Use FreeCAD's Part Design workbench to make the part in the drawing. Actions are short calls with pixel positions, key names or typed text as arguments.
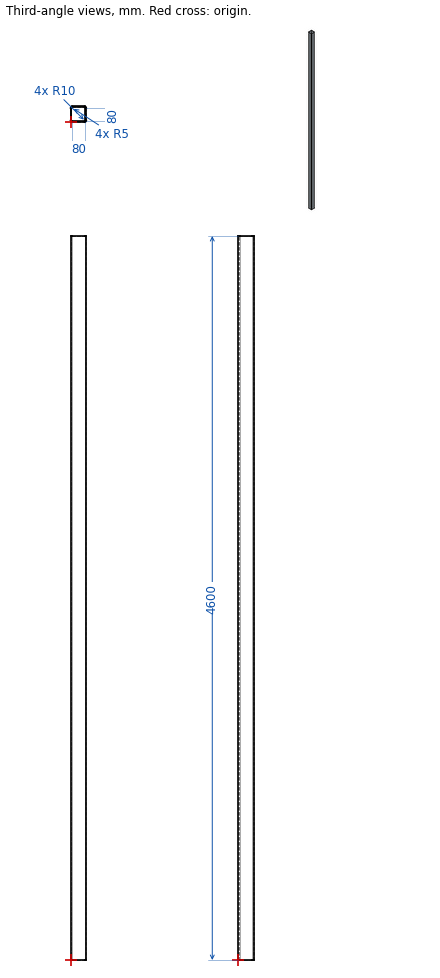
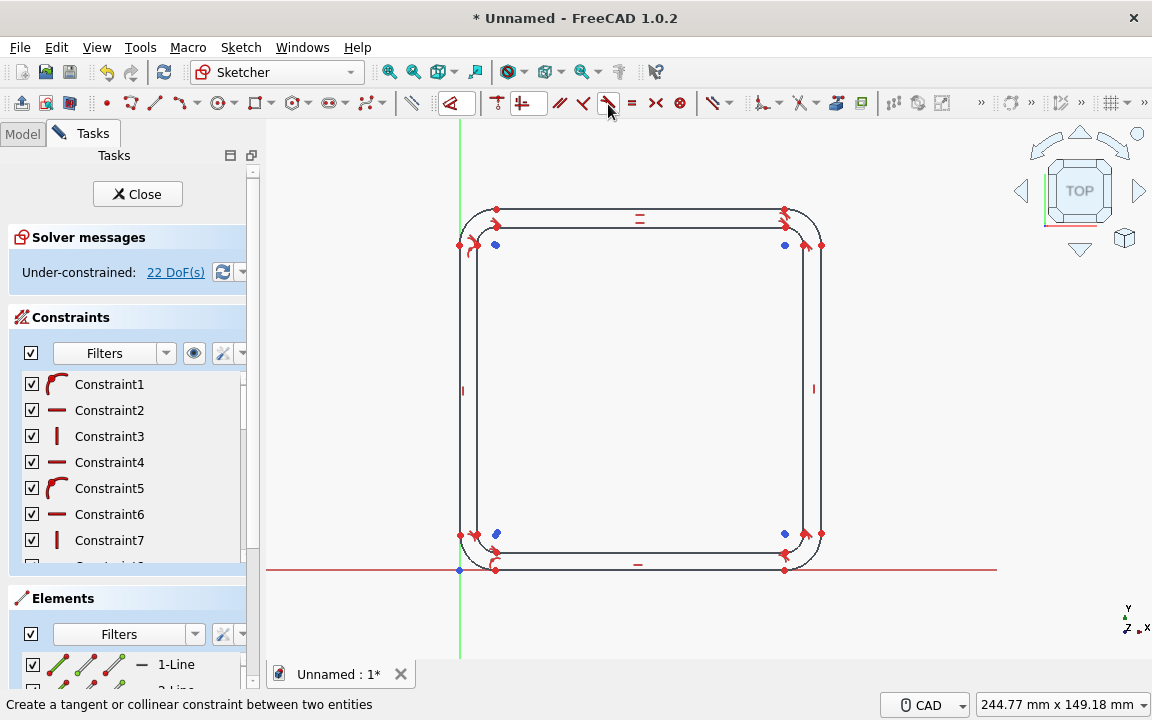
click(583, 228)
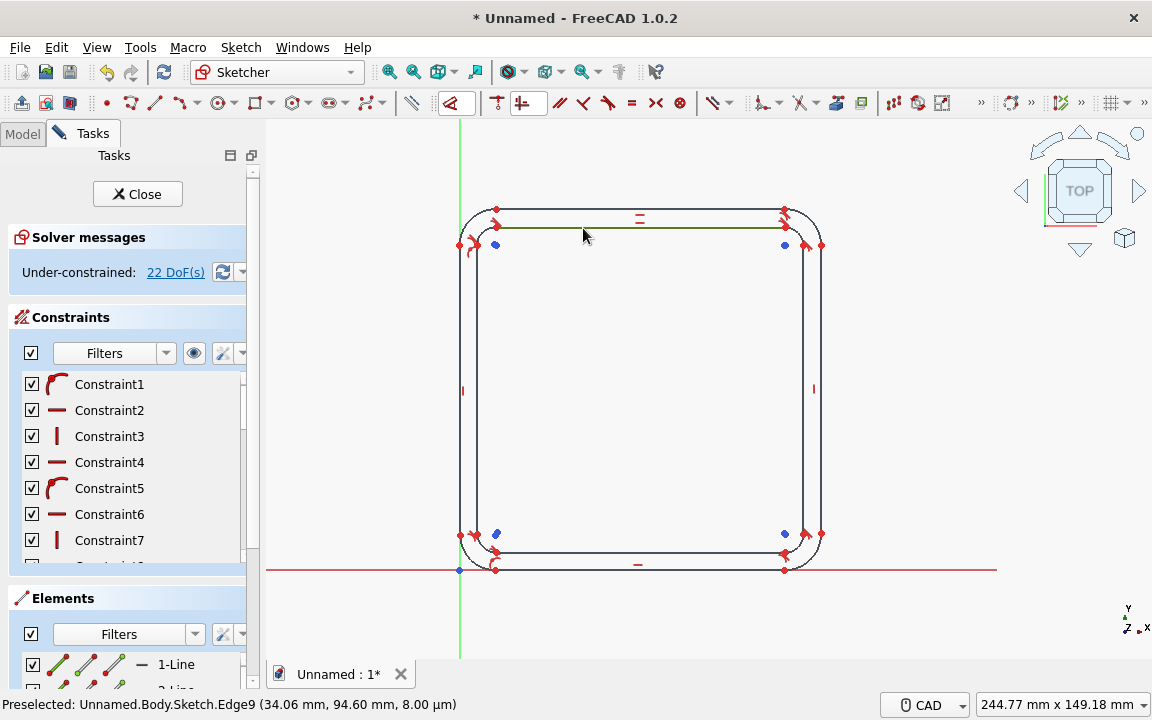
click(483, 232)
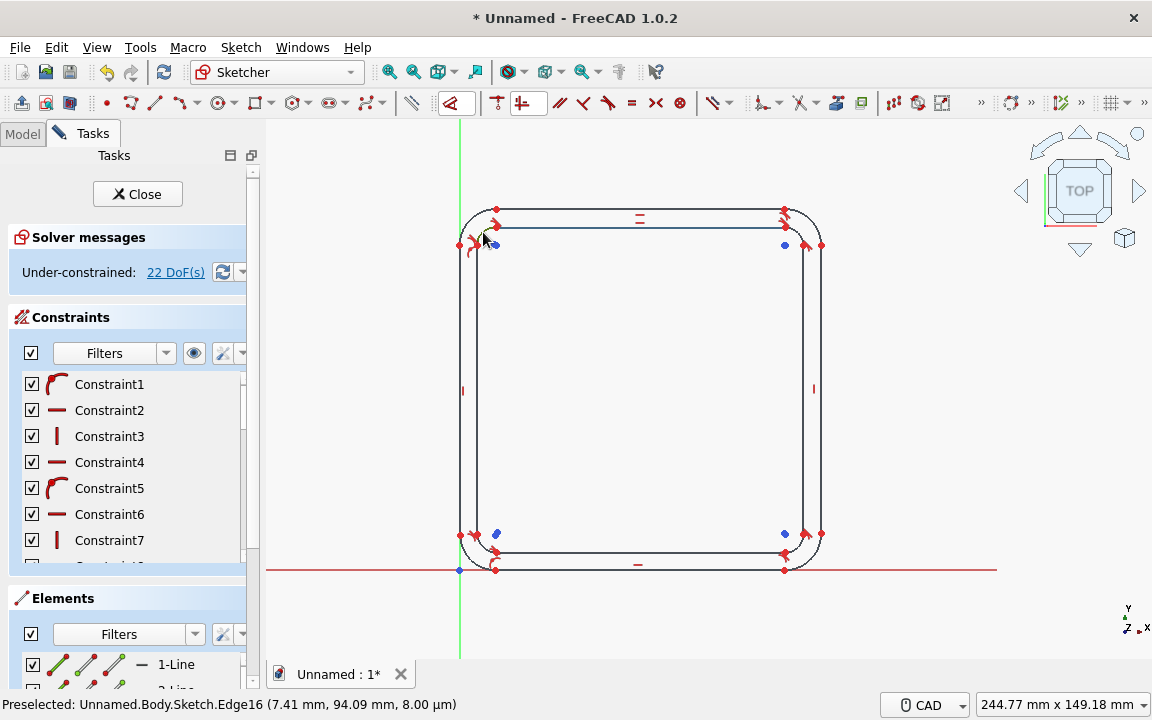
click(608, 104)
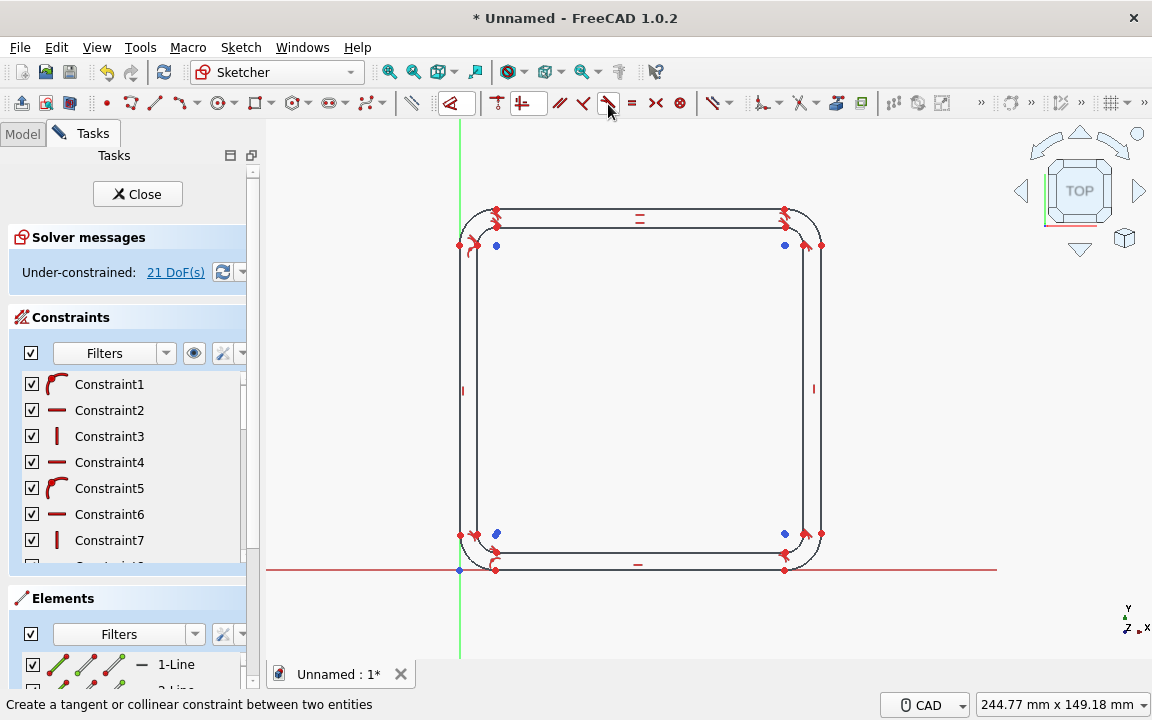
click(803, 332)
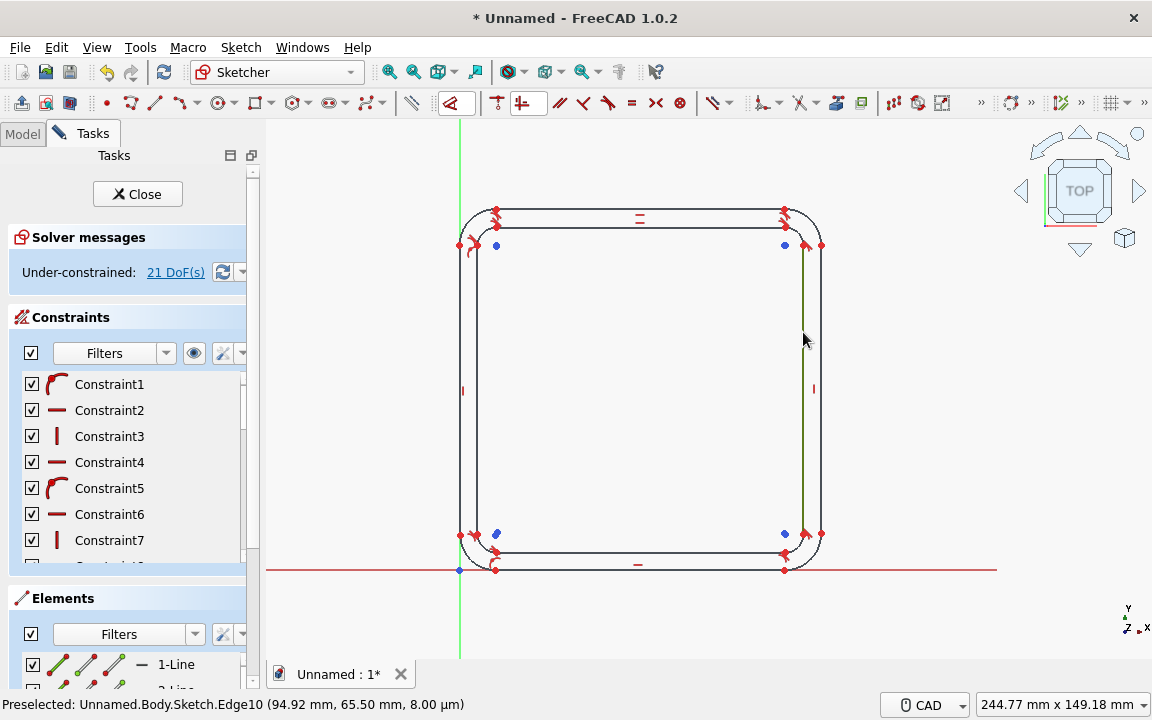
click(798, 233)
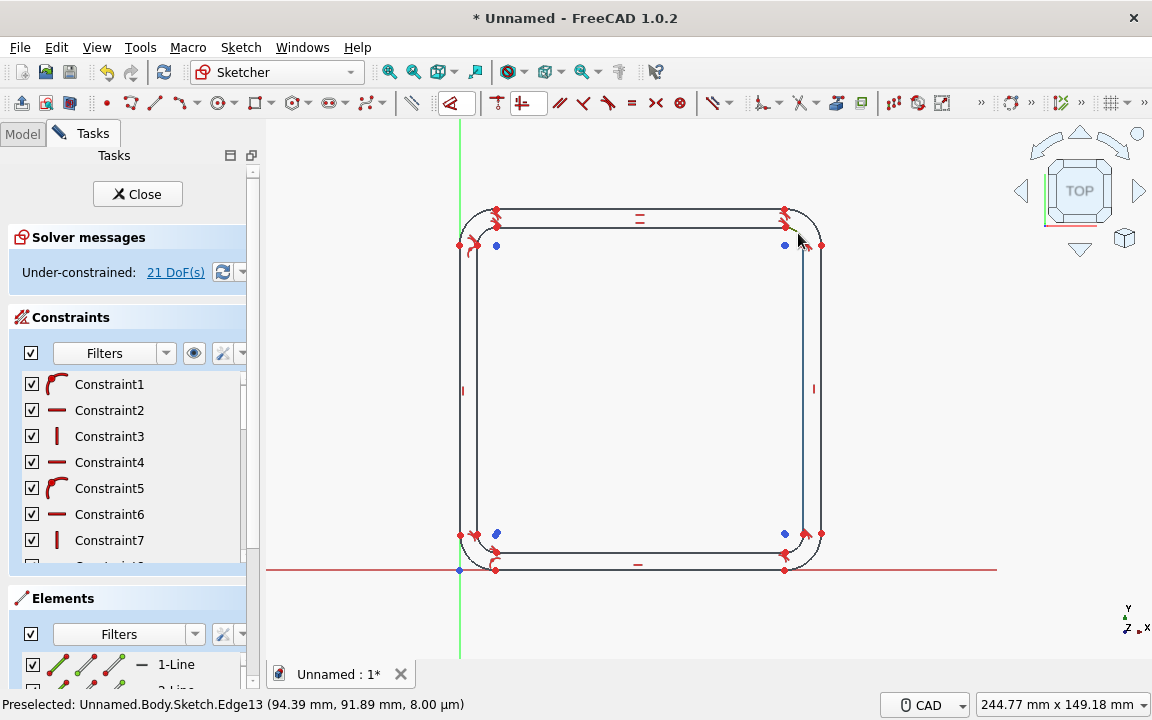
click(608, 104)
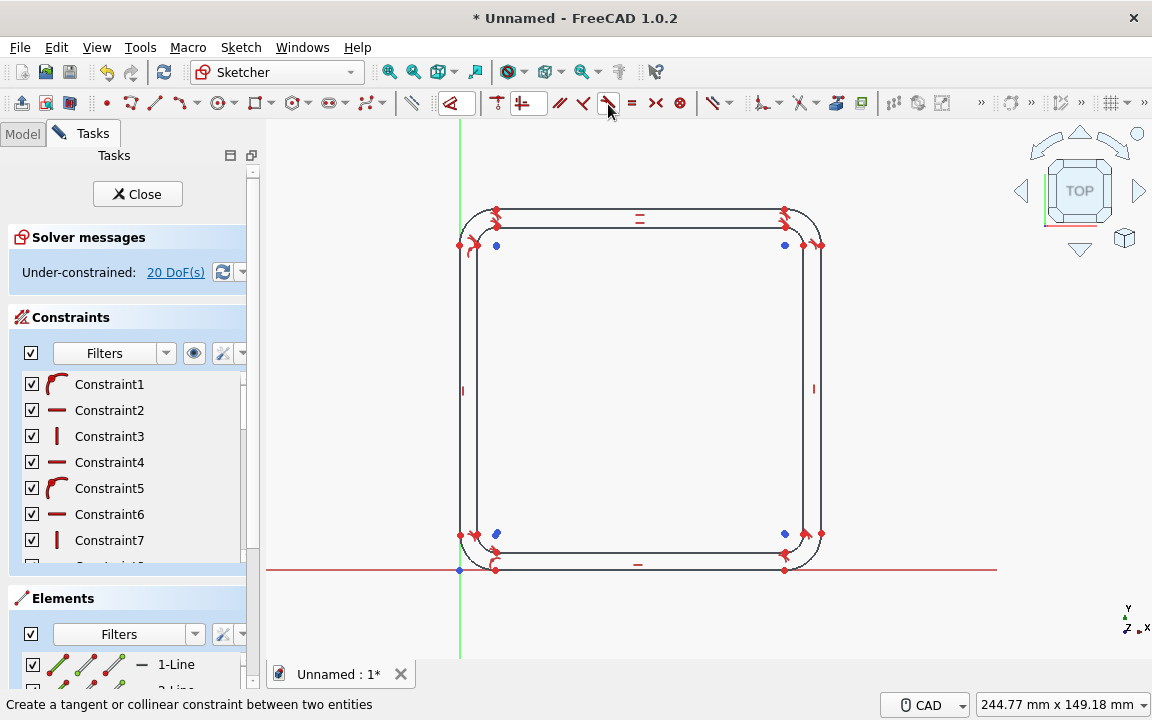
click(803, 332)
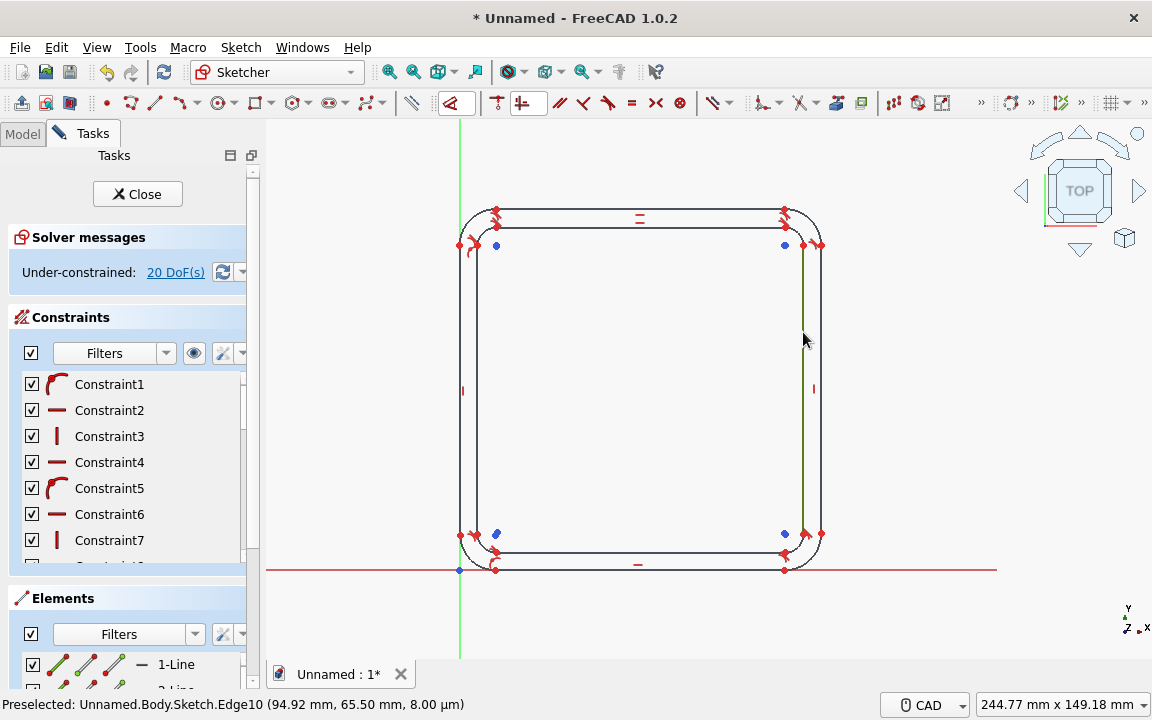
click(798, 547)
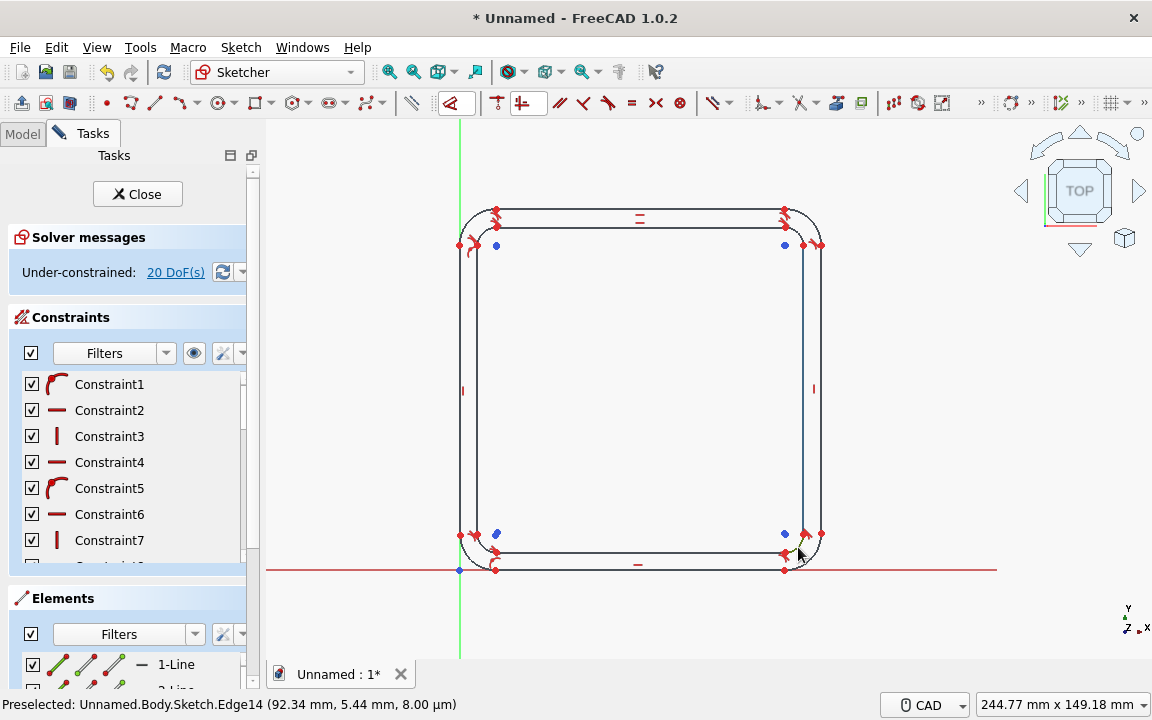
key(t)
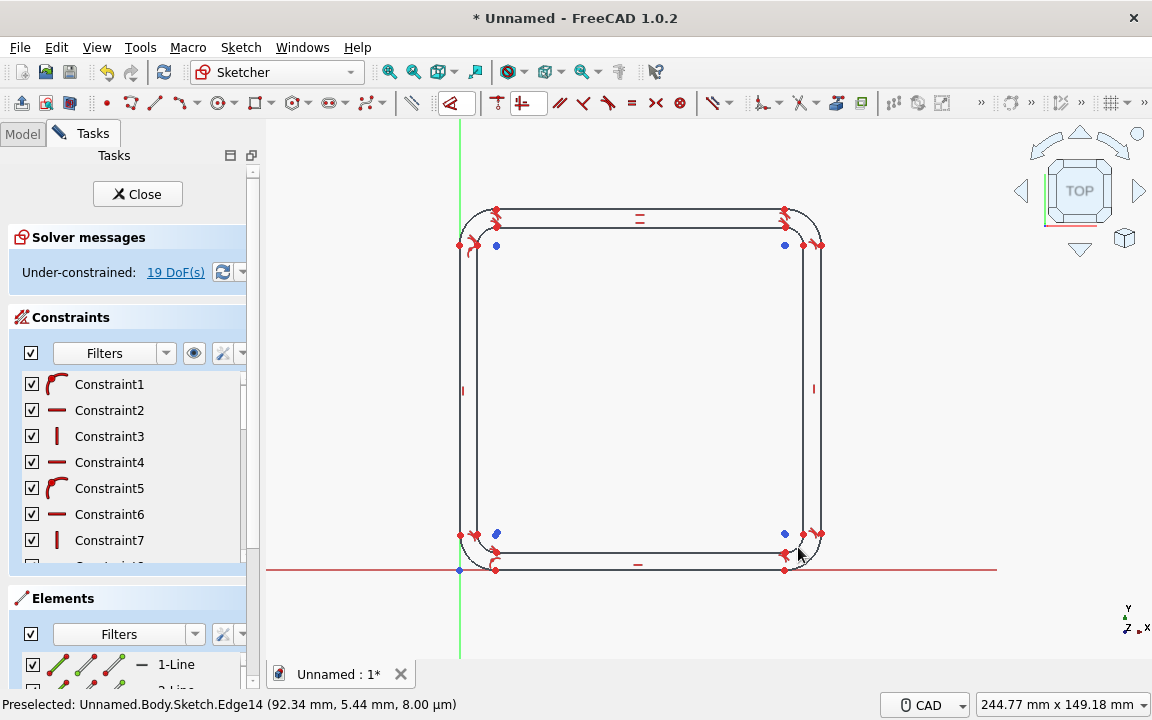
click(699, 553)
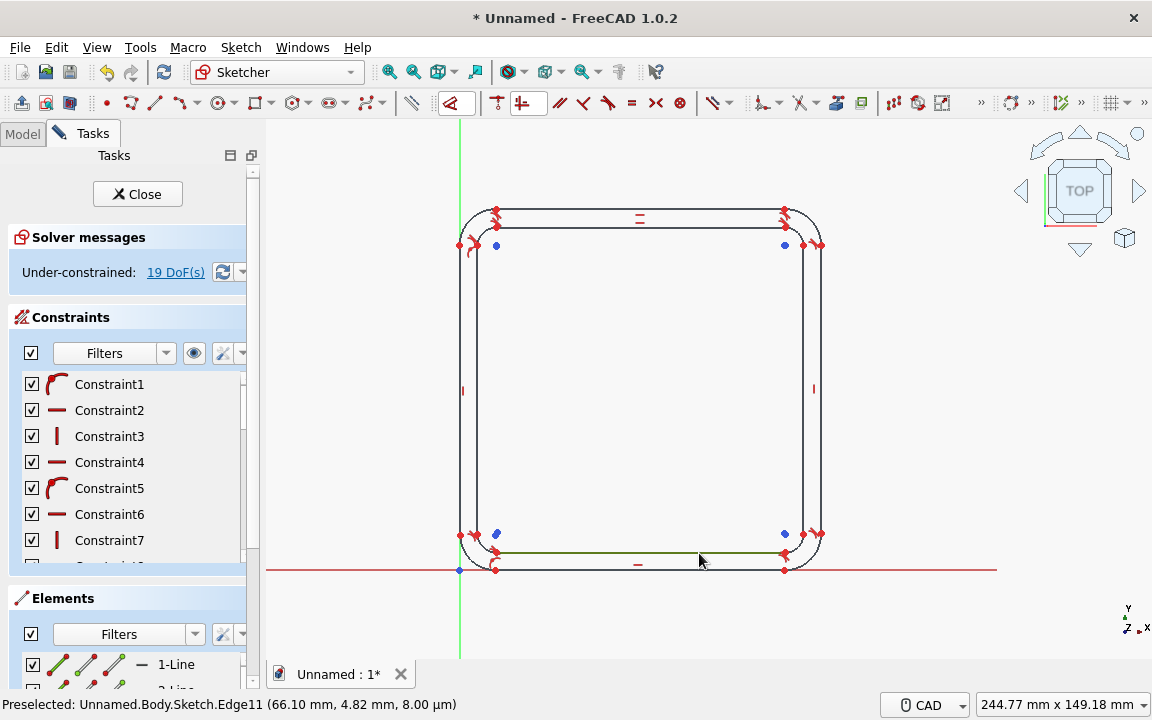
click(798, 547)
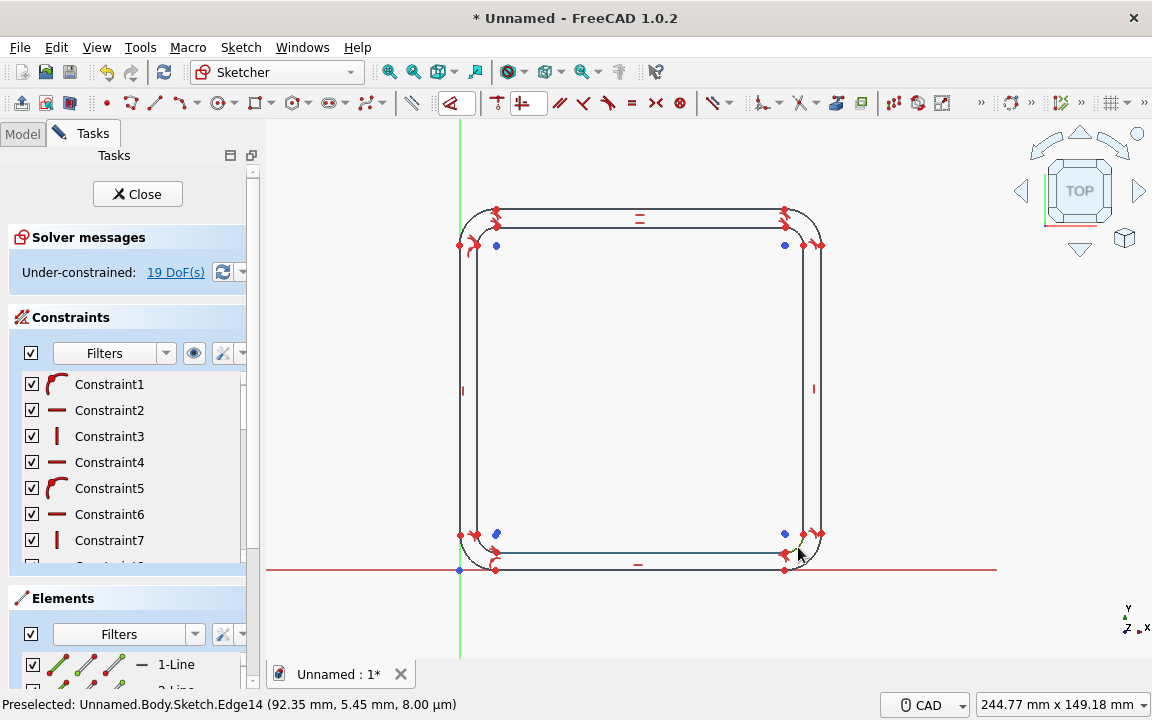
key(t)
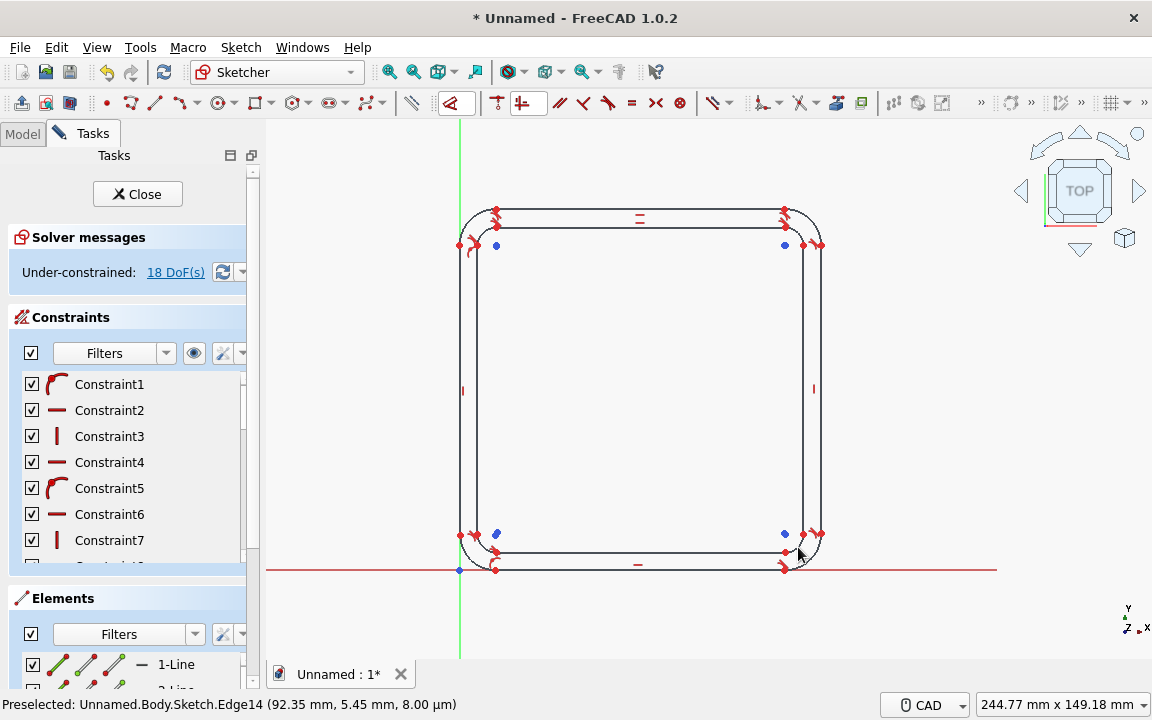
click(699, 553)